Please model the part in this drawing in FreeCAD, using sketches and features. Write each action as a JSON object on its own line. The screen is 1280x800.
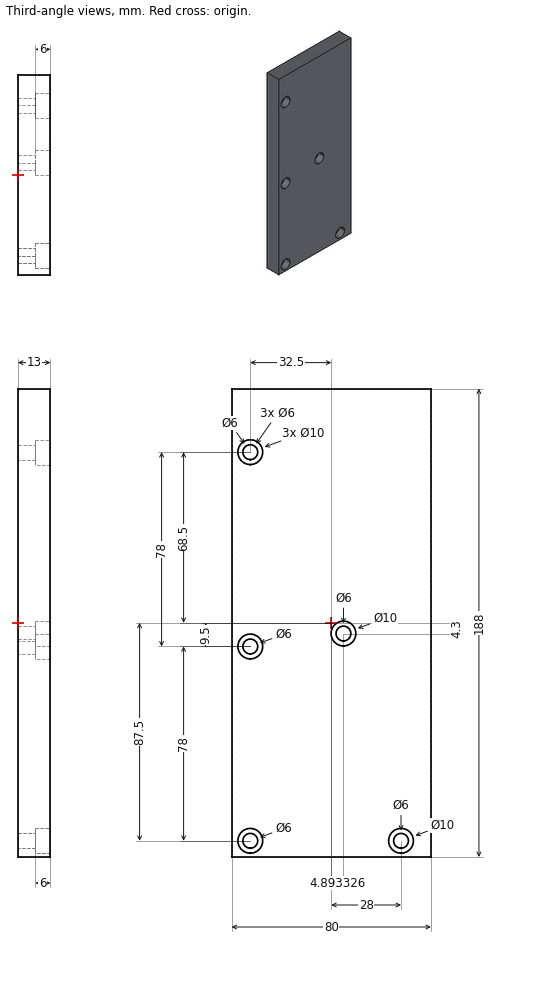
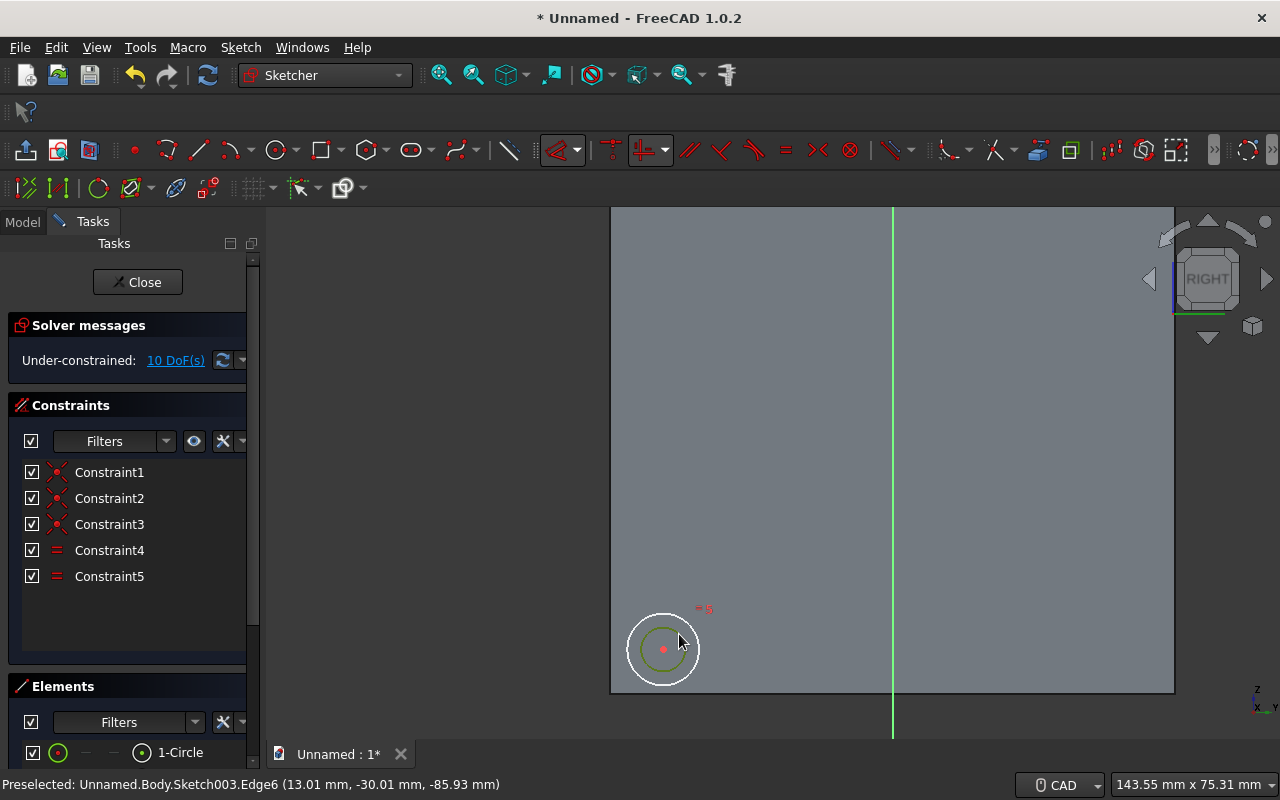
{"action": "left_click", "coordinate": [786, 150]}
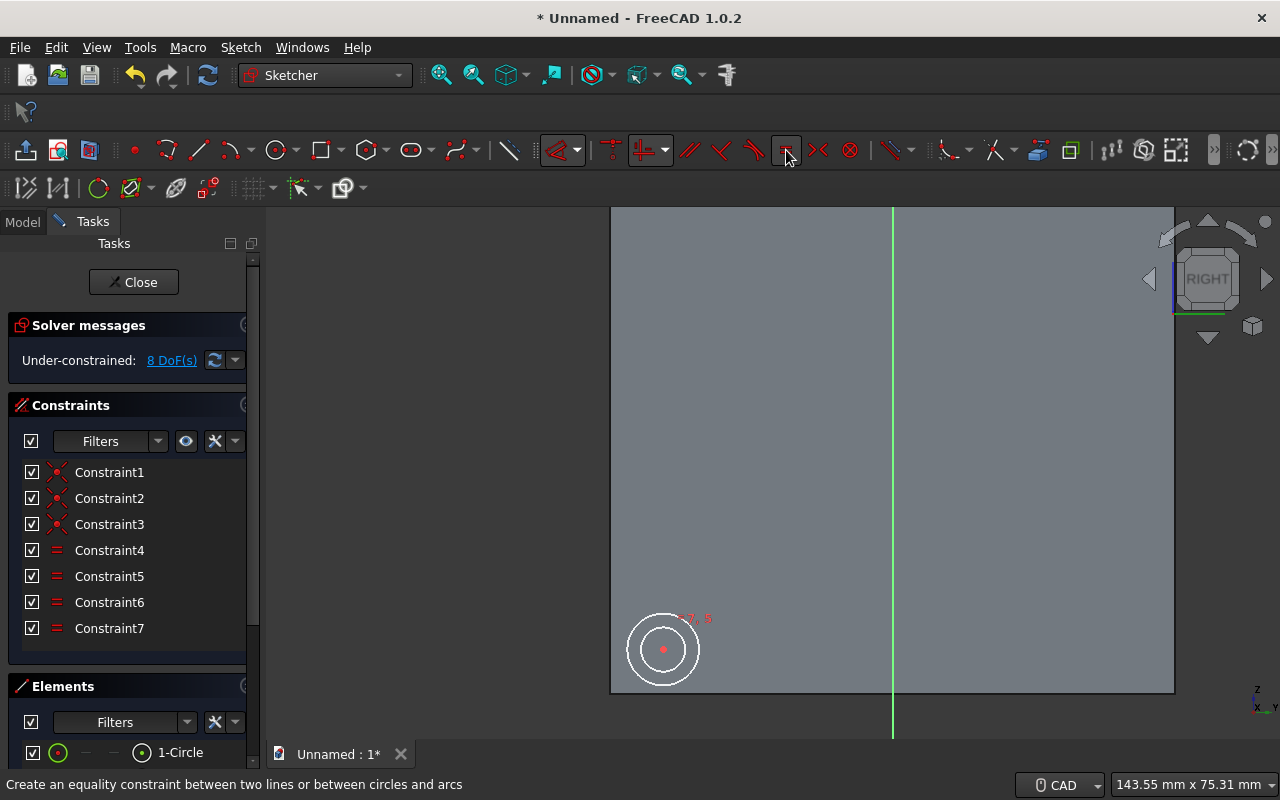
{"action": "scroll", "coordinate": [680, 635], "scroll_direction": "down", "scroll_amount": 6}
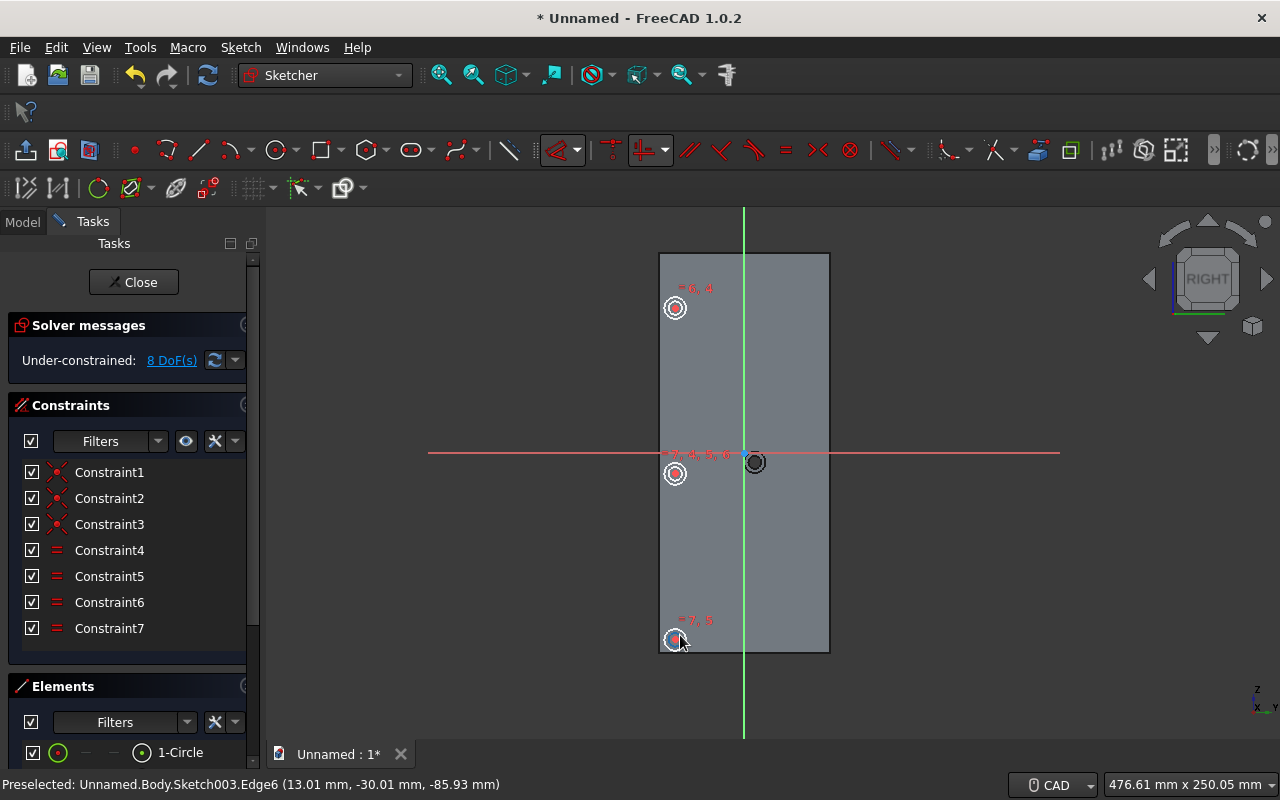
{"action": "scroll", "coordinate": [683, 300], "scroll_direction": "up", "scroll_amount": 7}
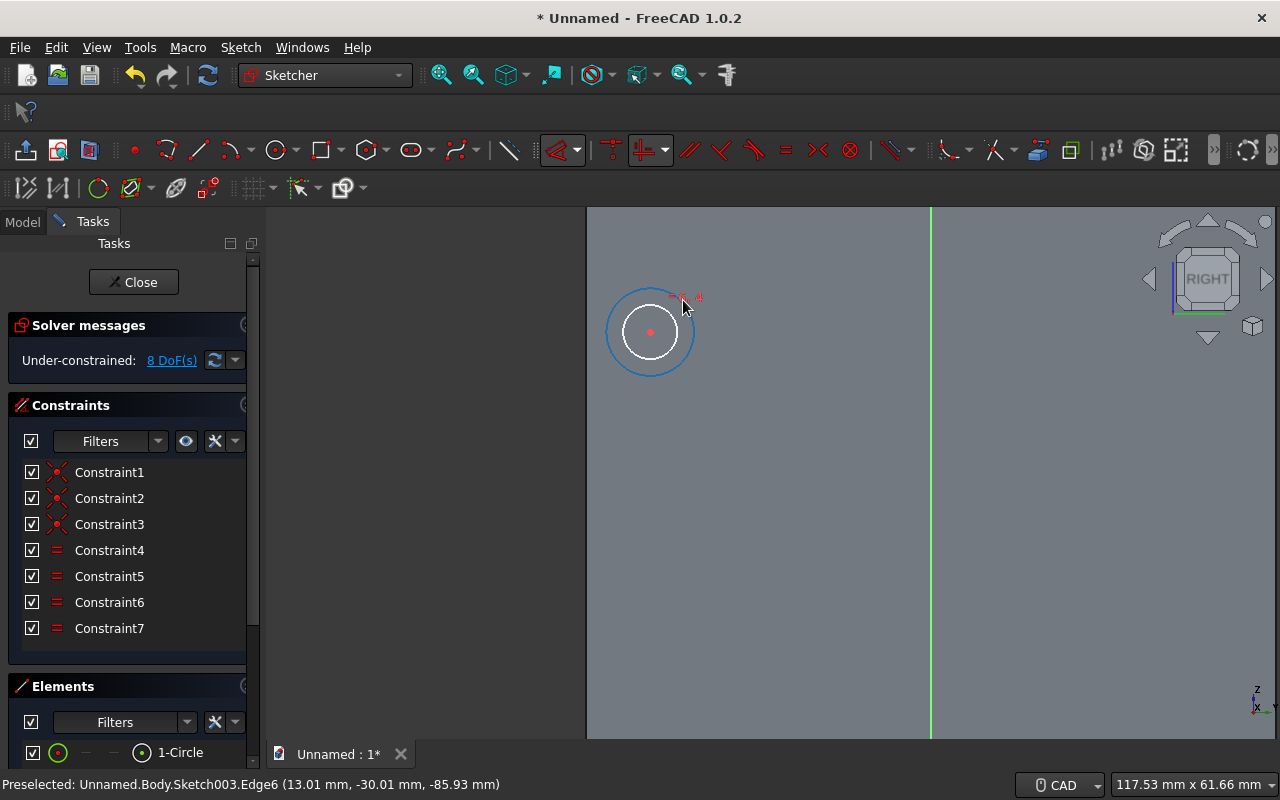
{"action": "left_click", "coordinate": [619, 301]}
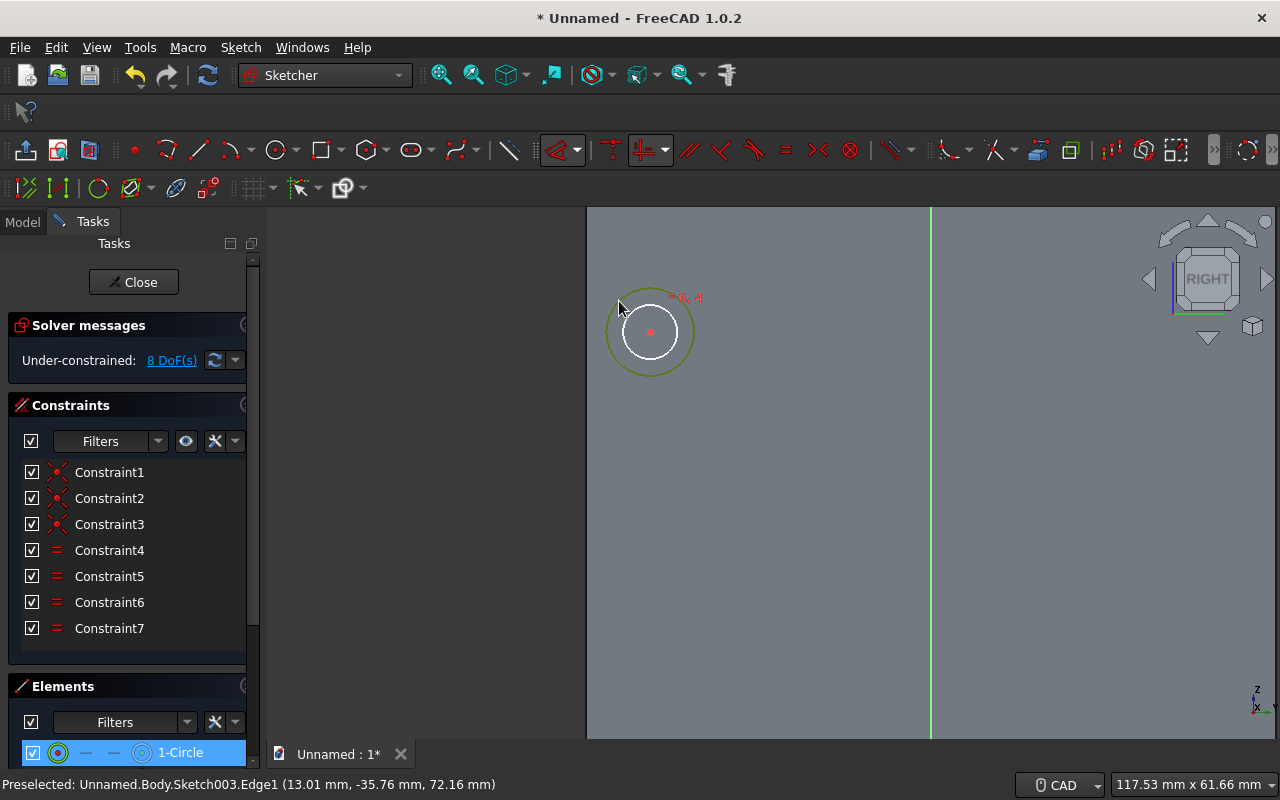
{"action": "key", "text": "k o"}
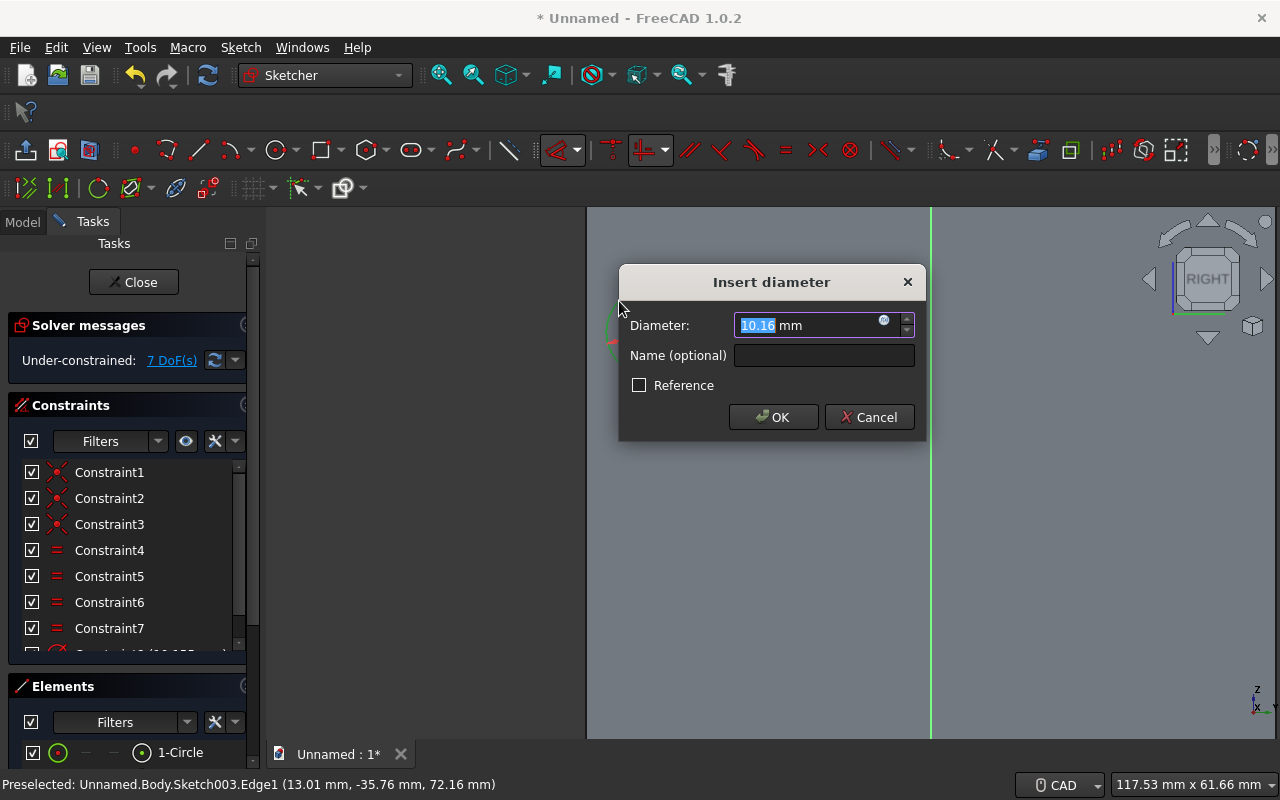
{"action": "type", "text": "10"}
{"action": "key", "text": "Return"}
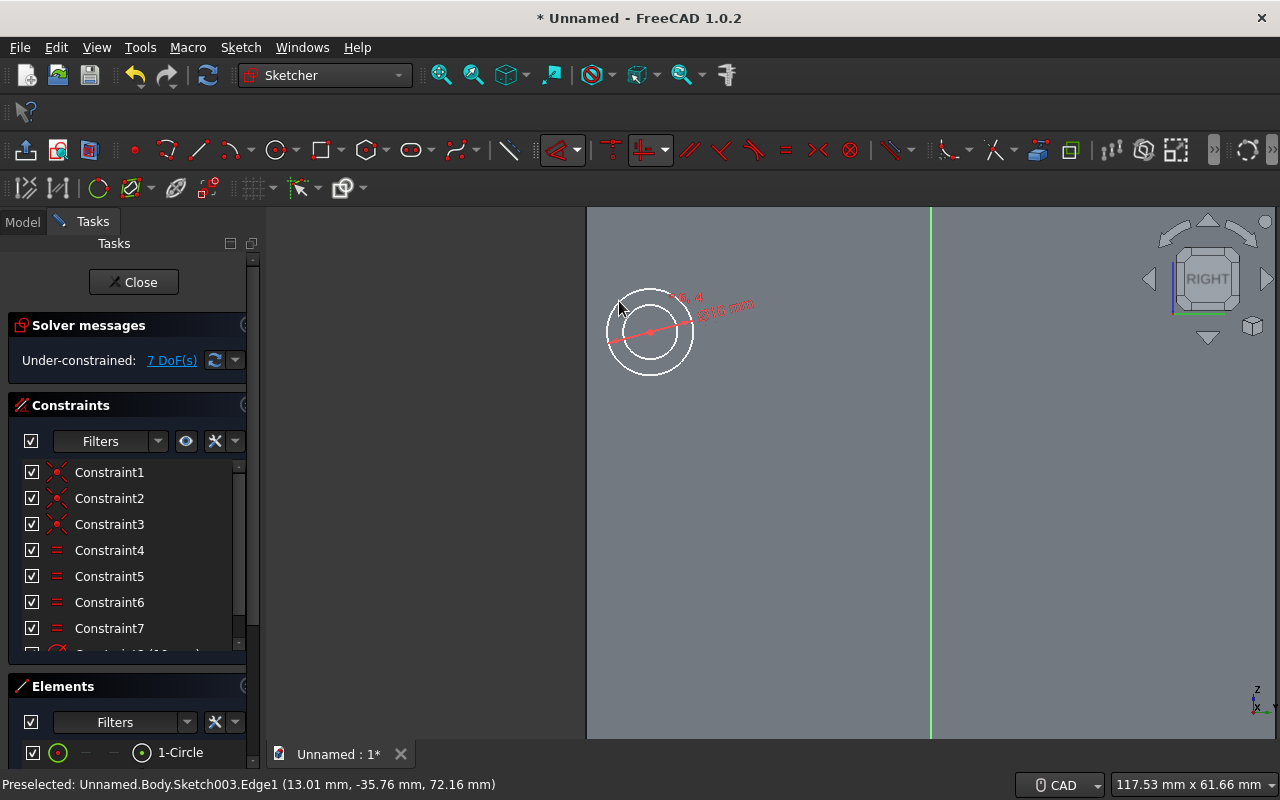
{"action": "left_click", "coordinate": [669, 313]}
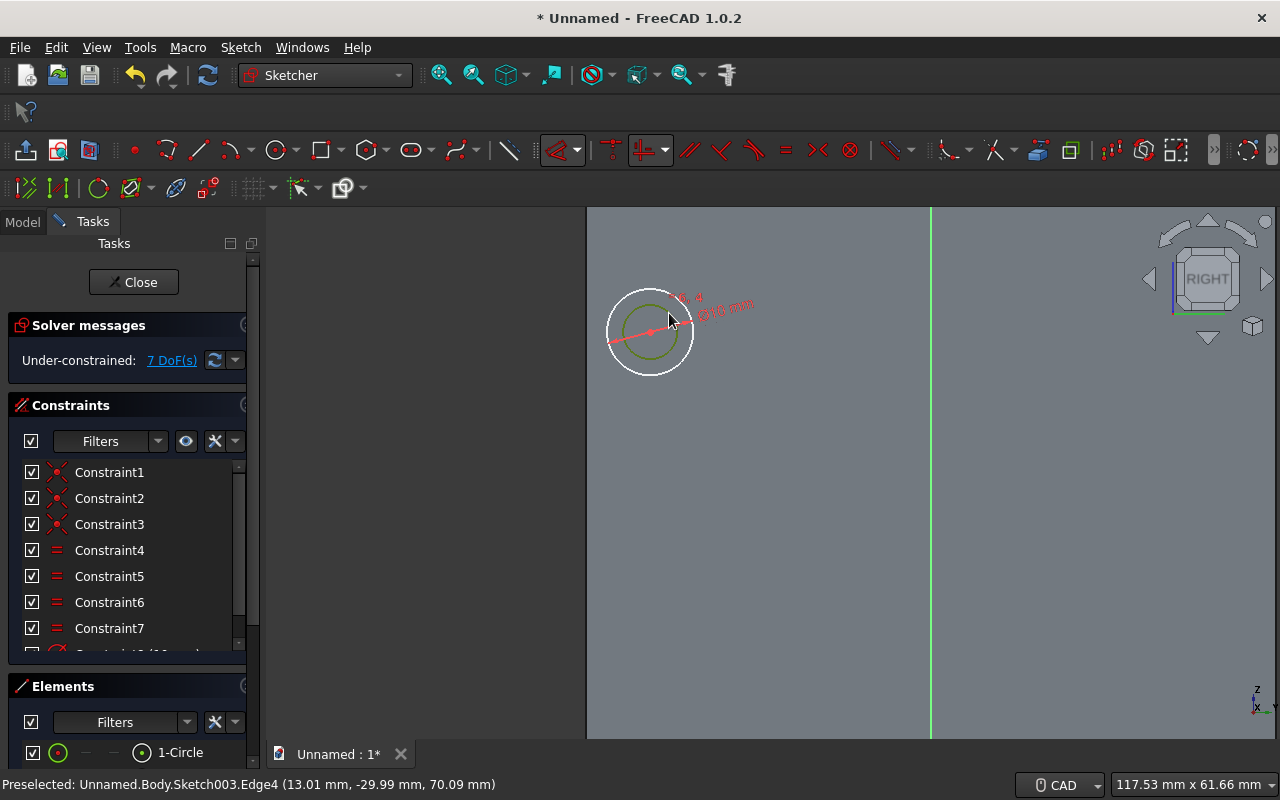
{"action": "left_click", "coordinate": [580, 150]}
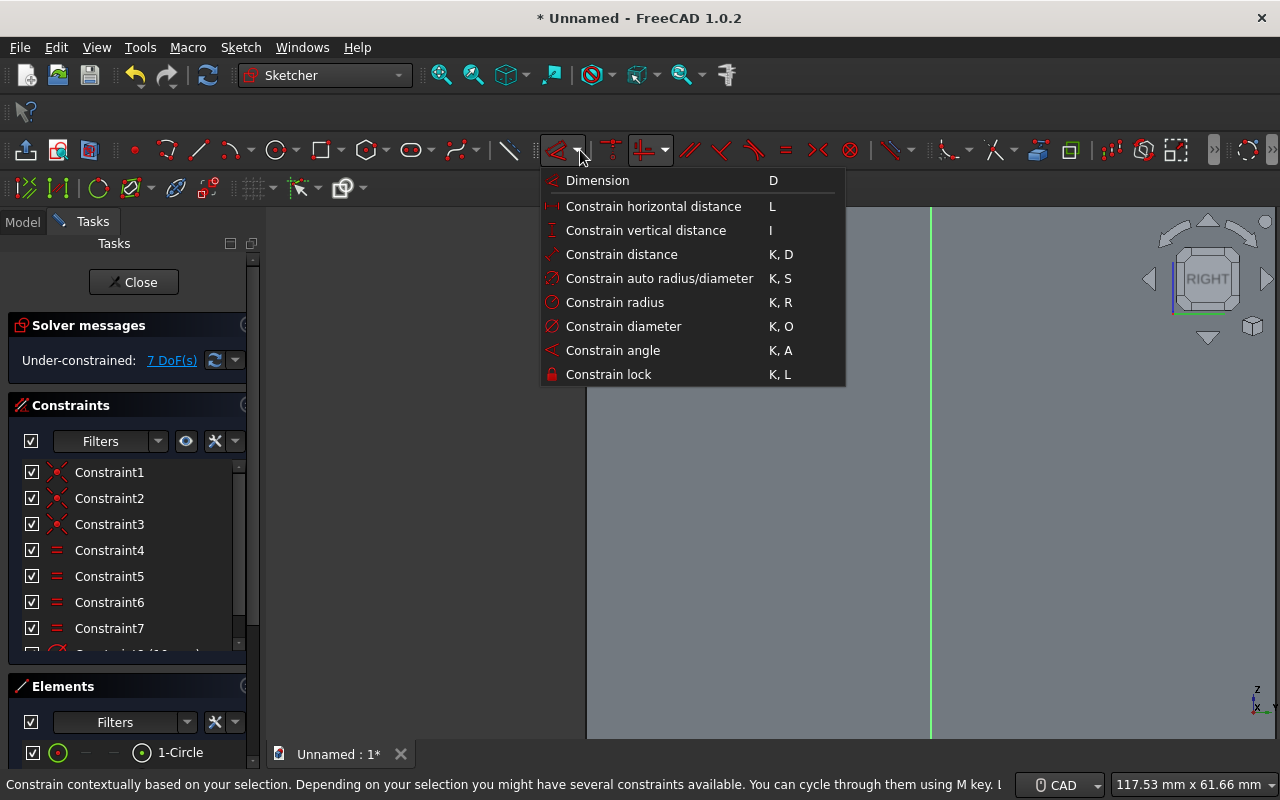
{"action": "left_click", "coordinate": [693, 326]}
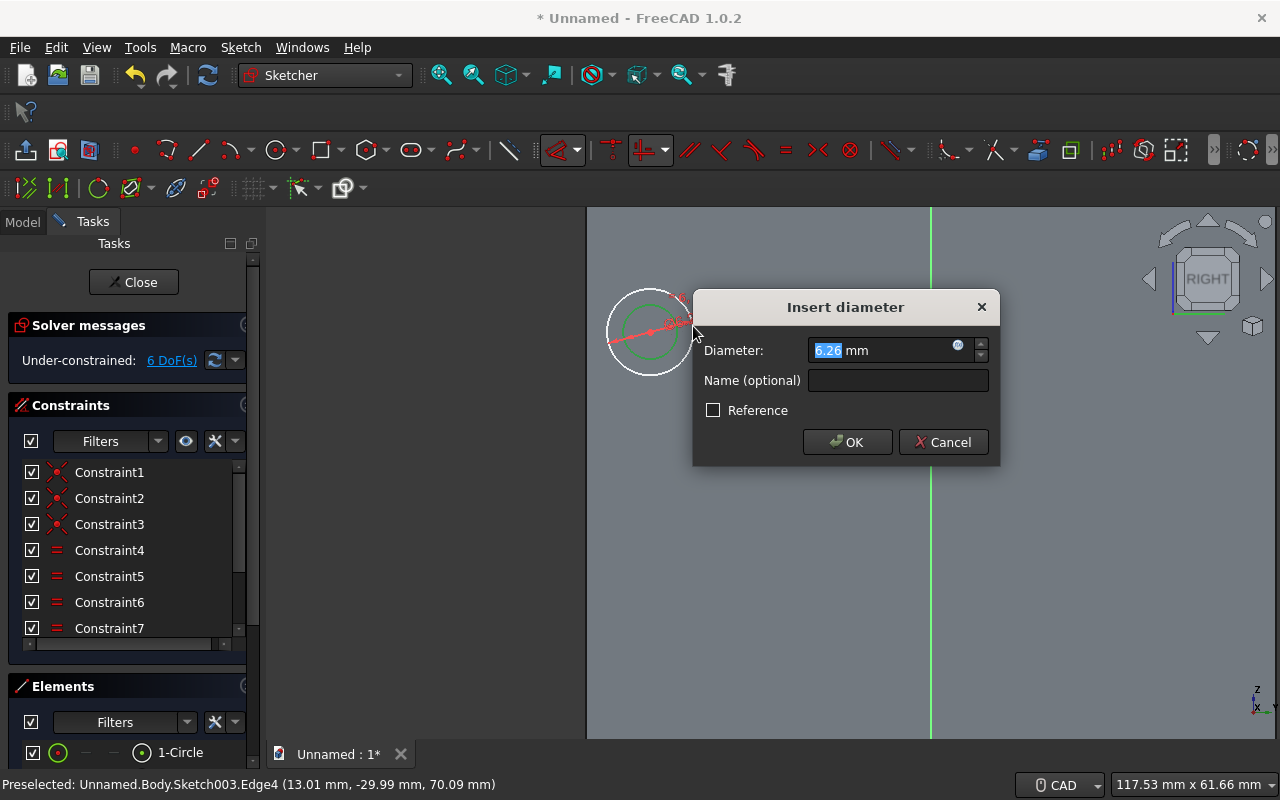
{"action": "type", "text": "6"}
{"action": "key", "text": "Return"}